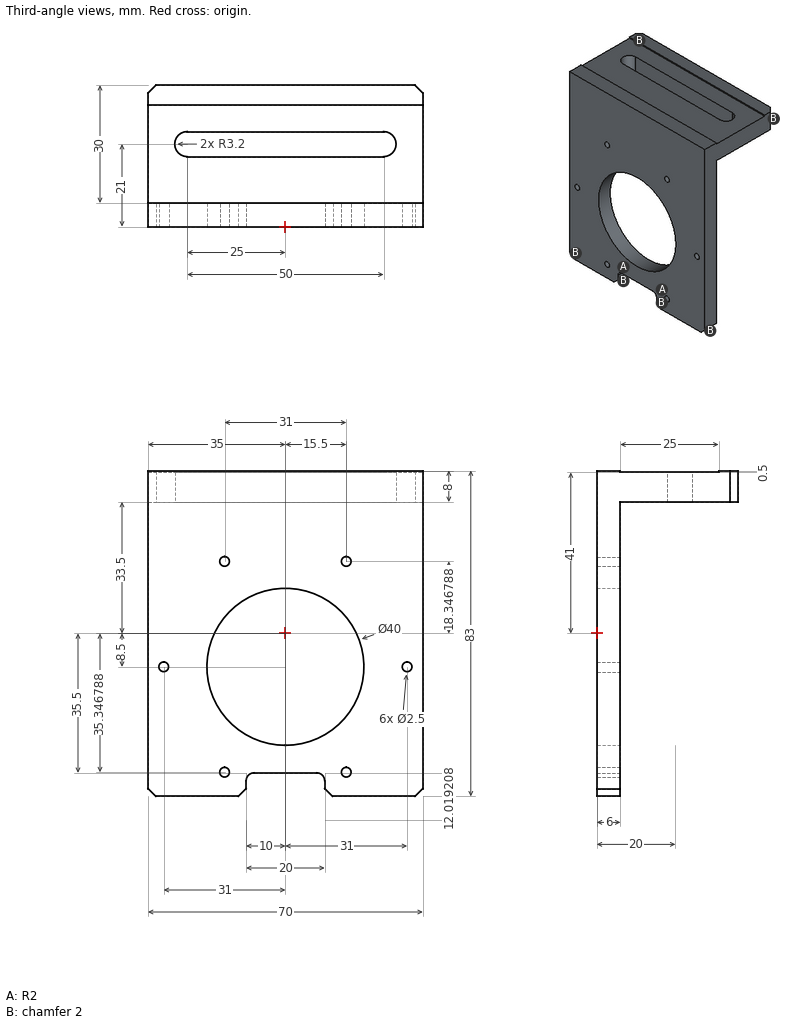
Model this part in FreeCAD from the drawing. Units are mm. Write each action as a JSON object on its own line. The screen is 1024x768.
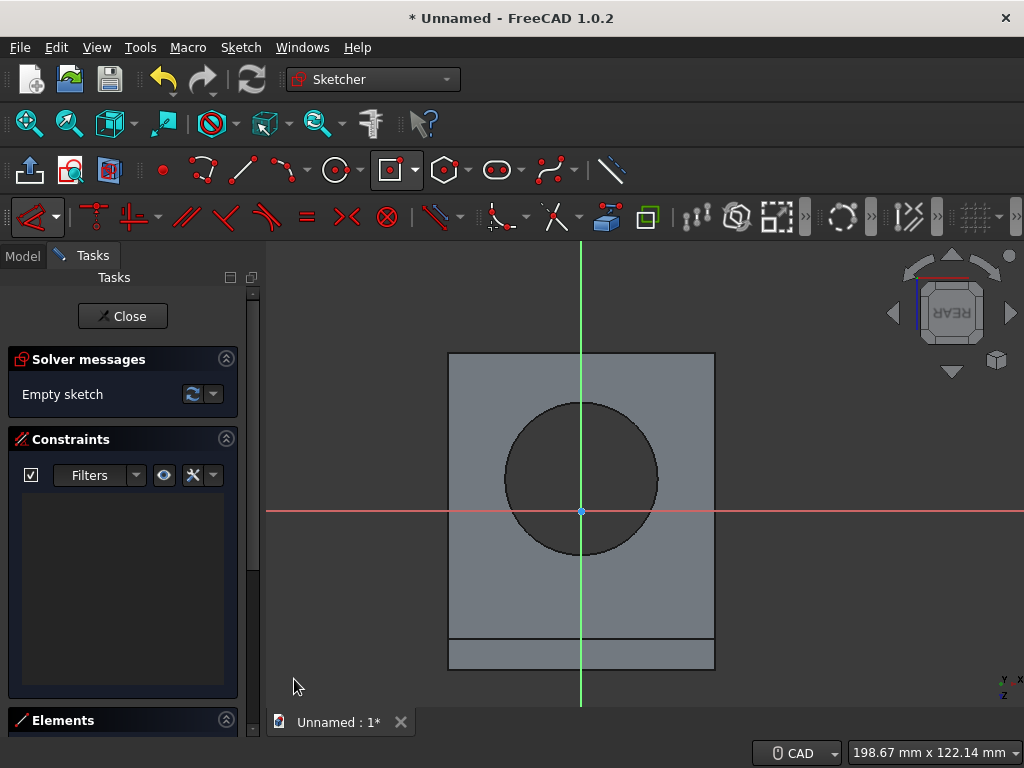
{"action": "scroll", "coordinate": [591, 312], "scroll_direction": "up", "scroll_amount": 2}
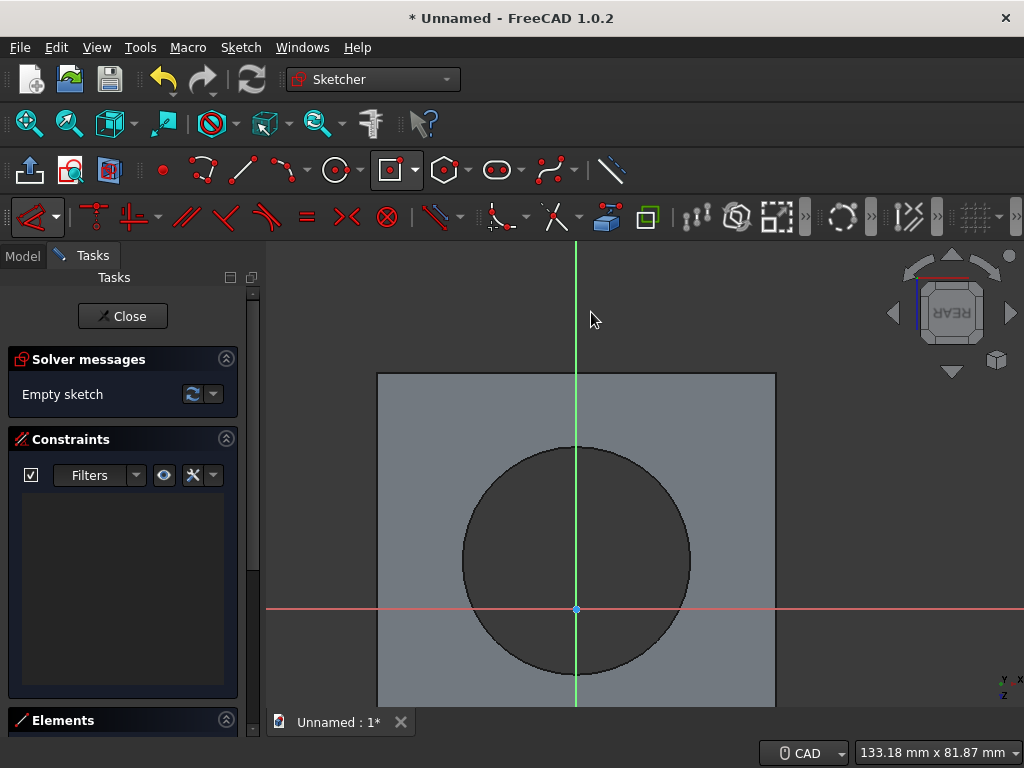
{"action": "left_click", "coordinate": [418, 170]}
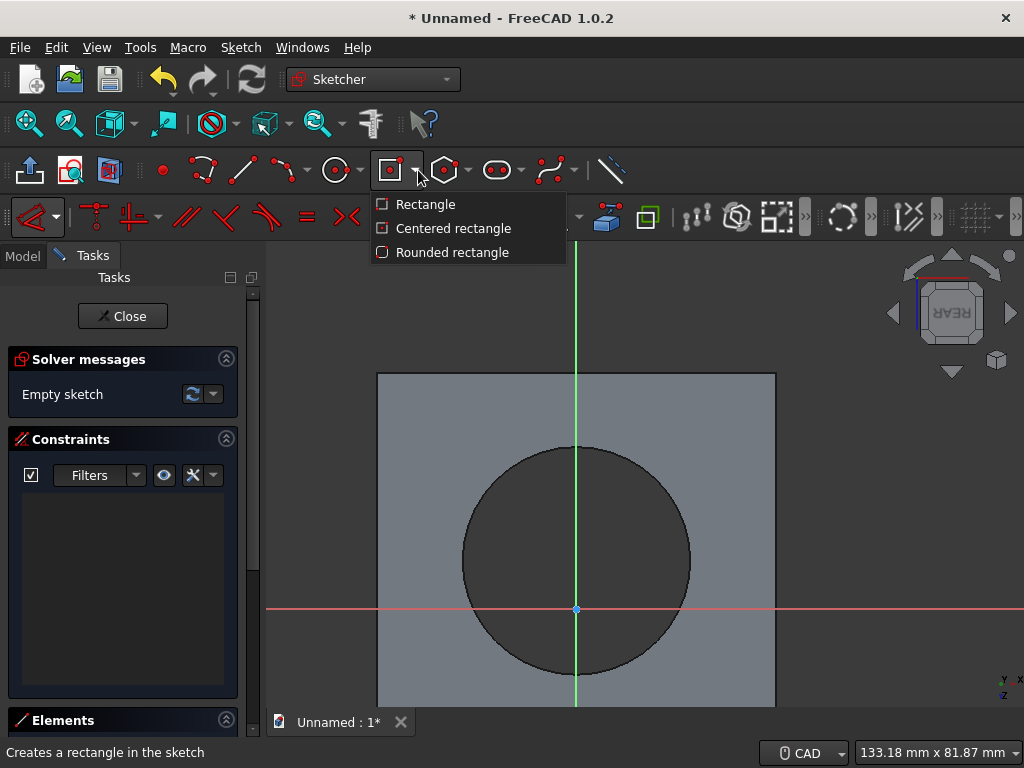
{"action": "left_click", "coordinate": [468, 204]}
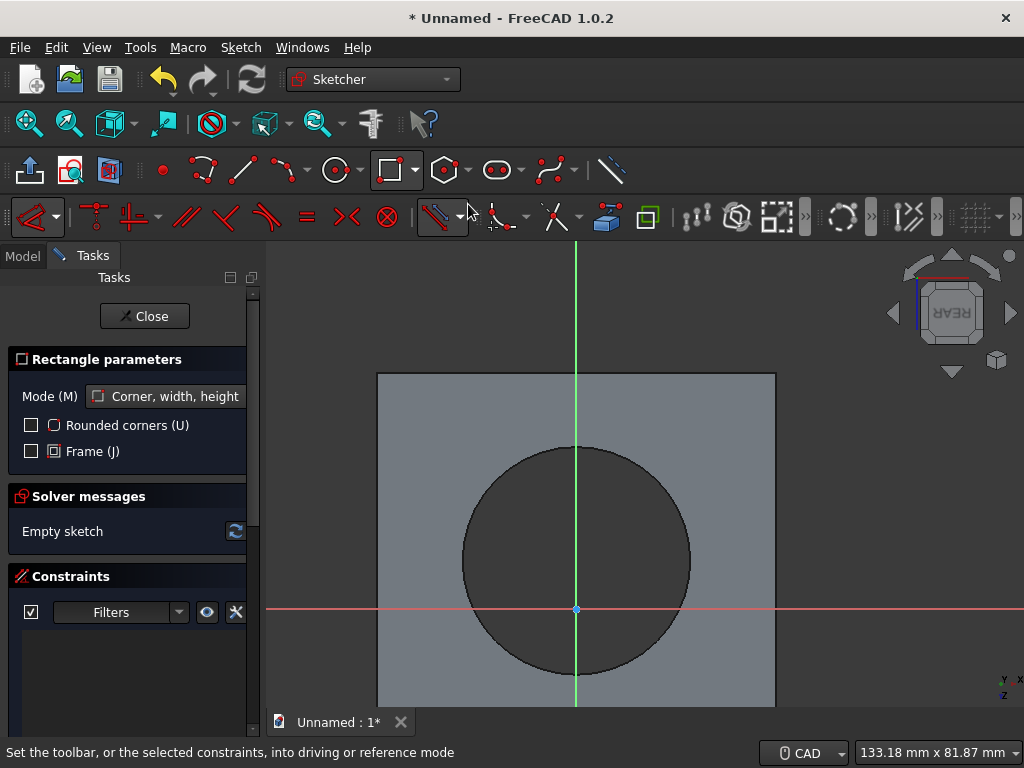
{"action": "left_click", "coordinate": [520, 339]}
{"action": "mouse_move", "coordinate": [633, 407]}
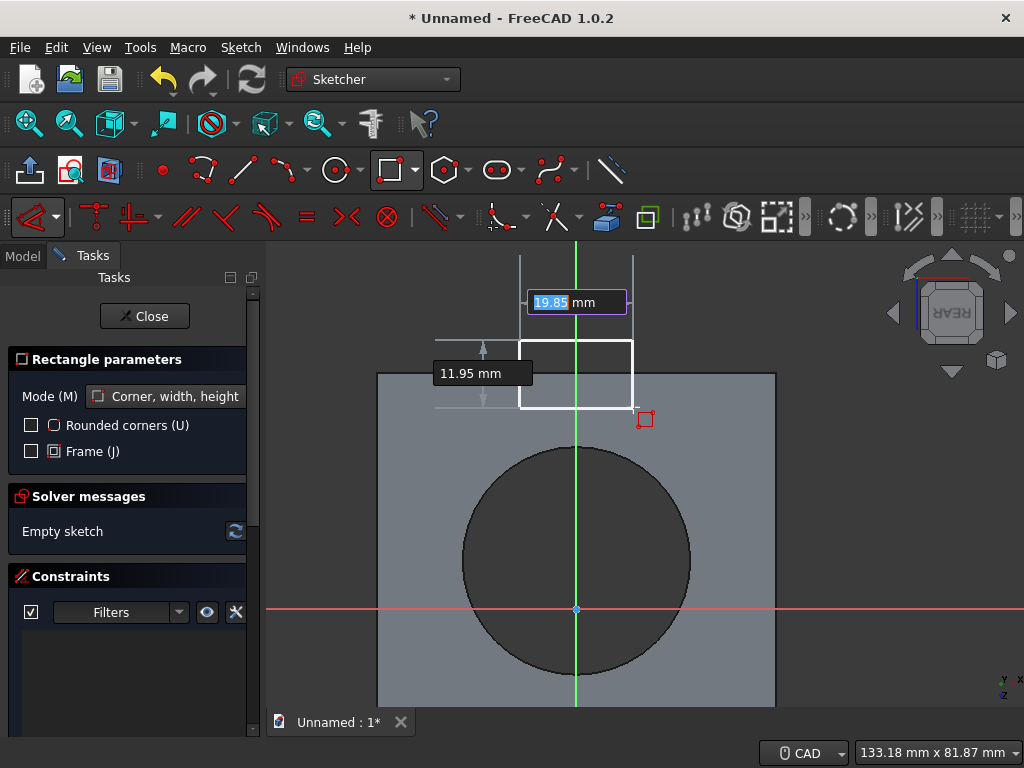
{"action": "type", "text": "20"}
{"action": "key", "text": "Tab"}
{"action": "type", "text": "12.019208"}
{"action": "key", "text": "Return"}
{"action": "key", "text": "Escape"}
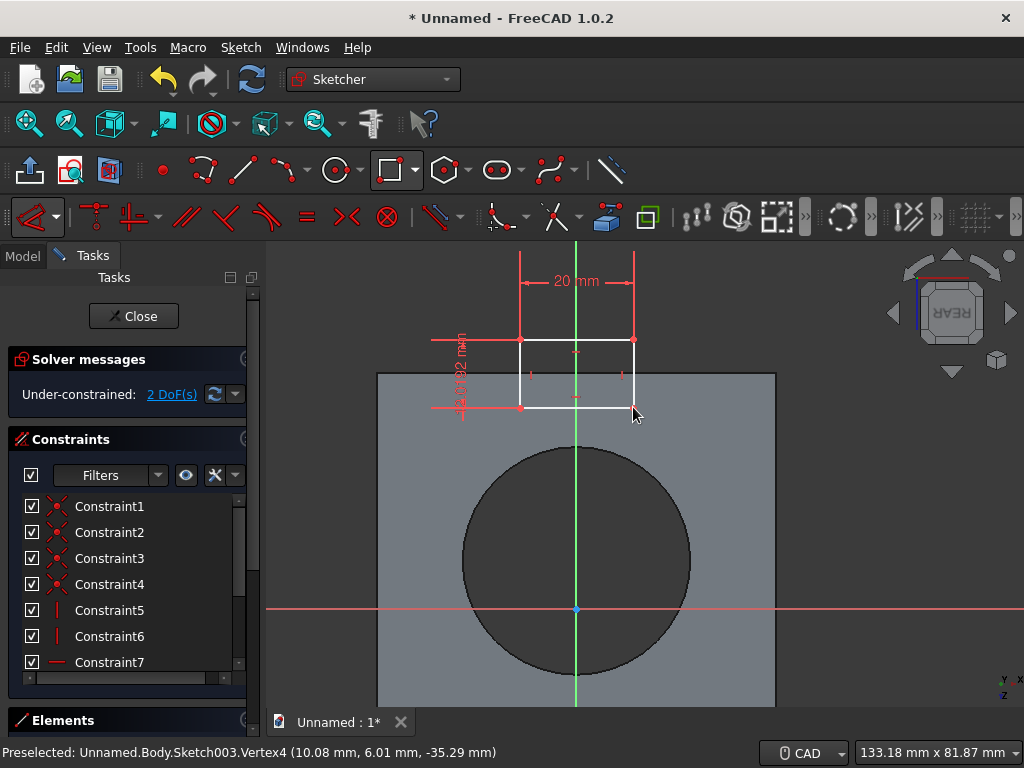
{"action": "left_click", "coordinate": [520, 340]}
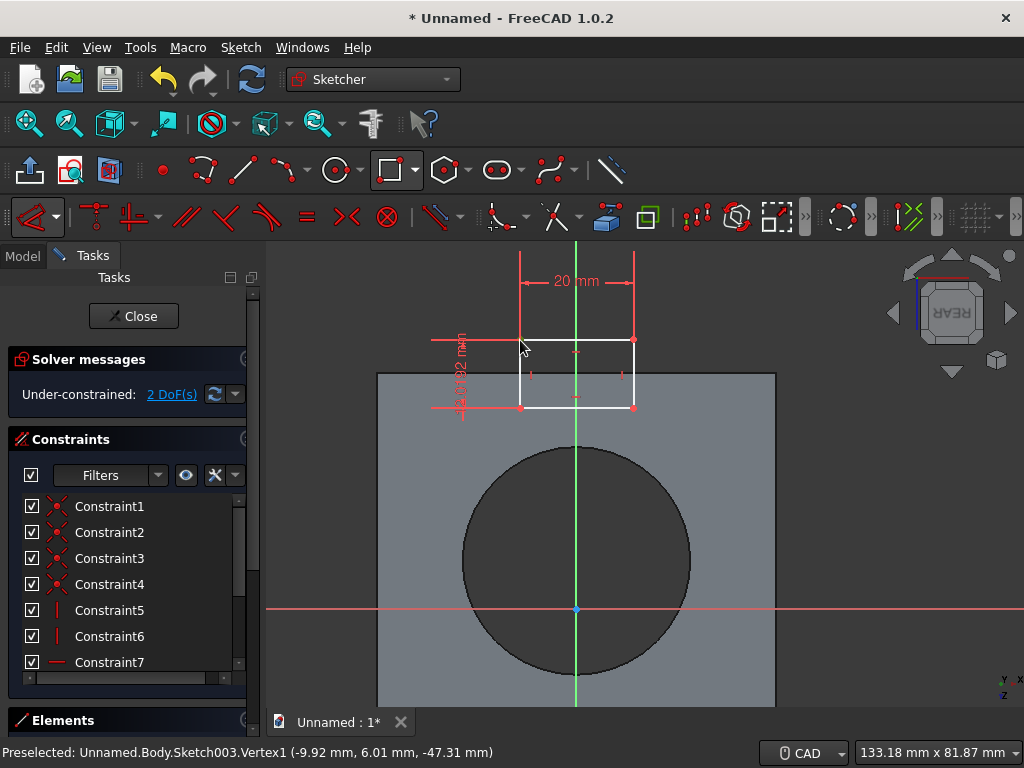
{"action": "key", "text": "l"}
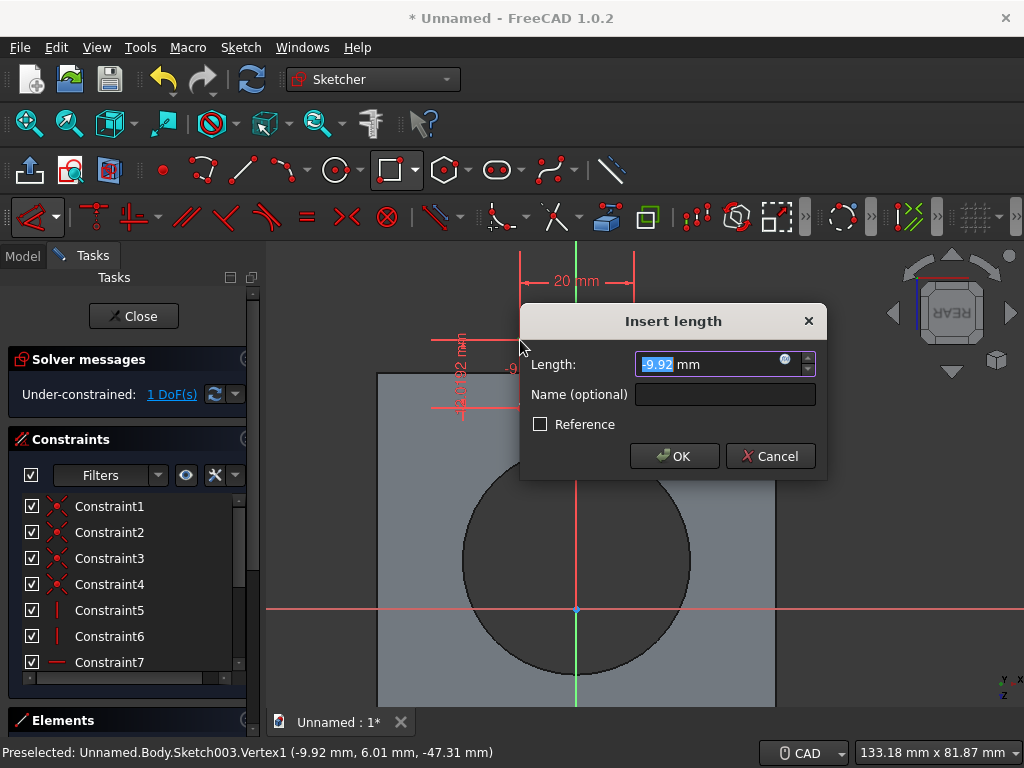
{"action": "type", "text": "-10"}
{"action": "key", "text": "Return"}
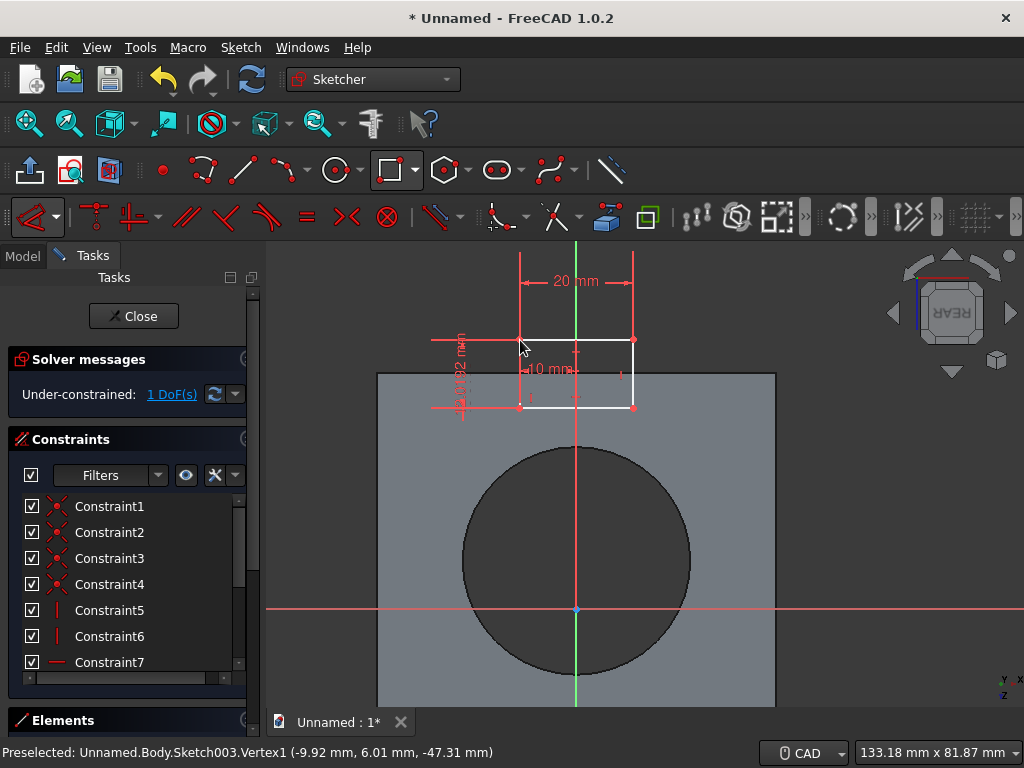
{"action": "left_click", "coordinate": [520, 408]}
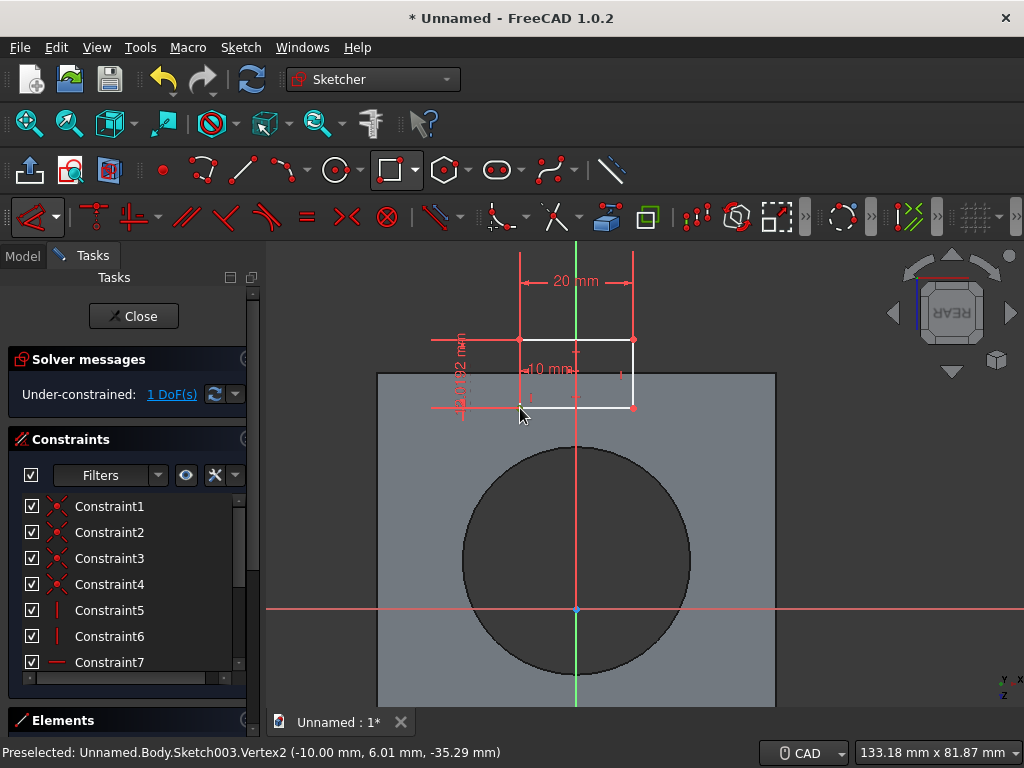
{"action": "left_click", "coordinate": [58, 218]}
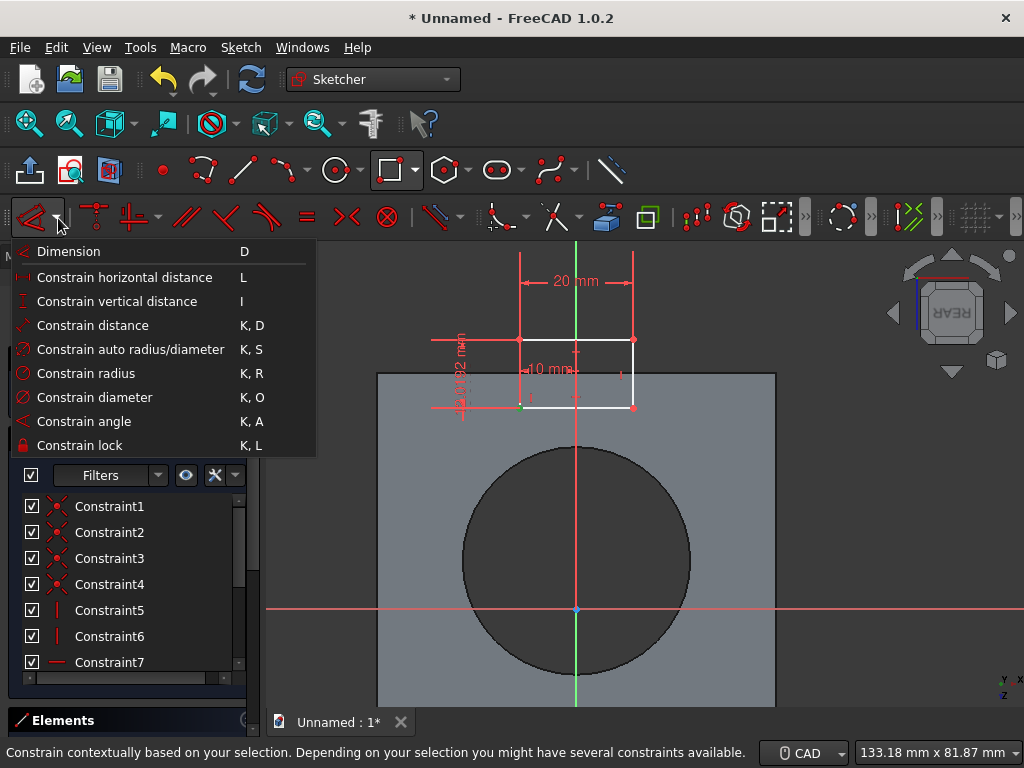
{"action": "left_click", "coordinate": [164, 301]}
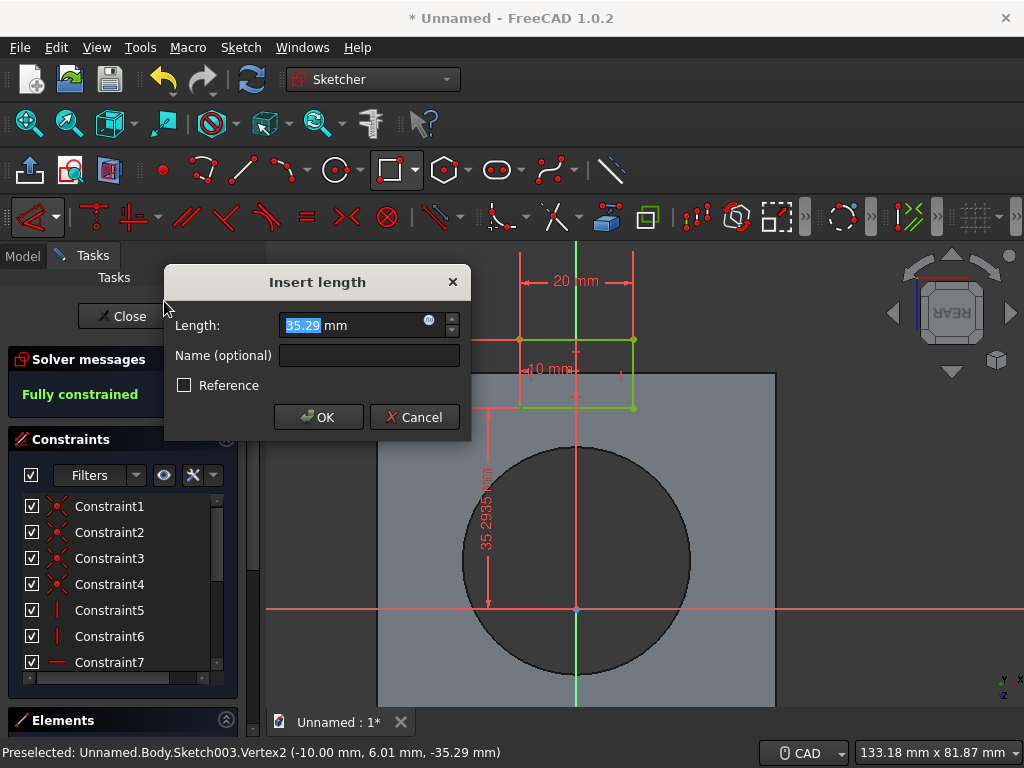
{"action": "type", "text": "35.5"}
{"action": "key", "text": "Return"}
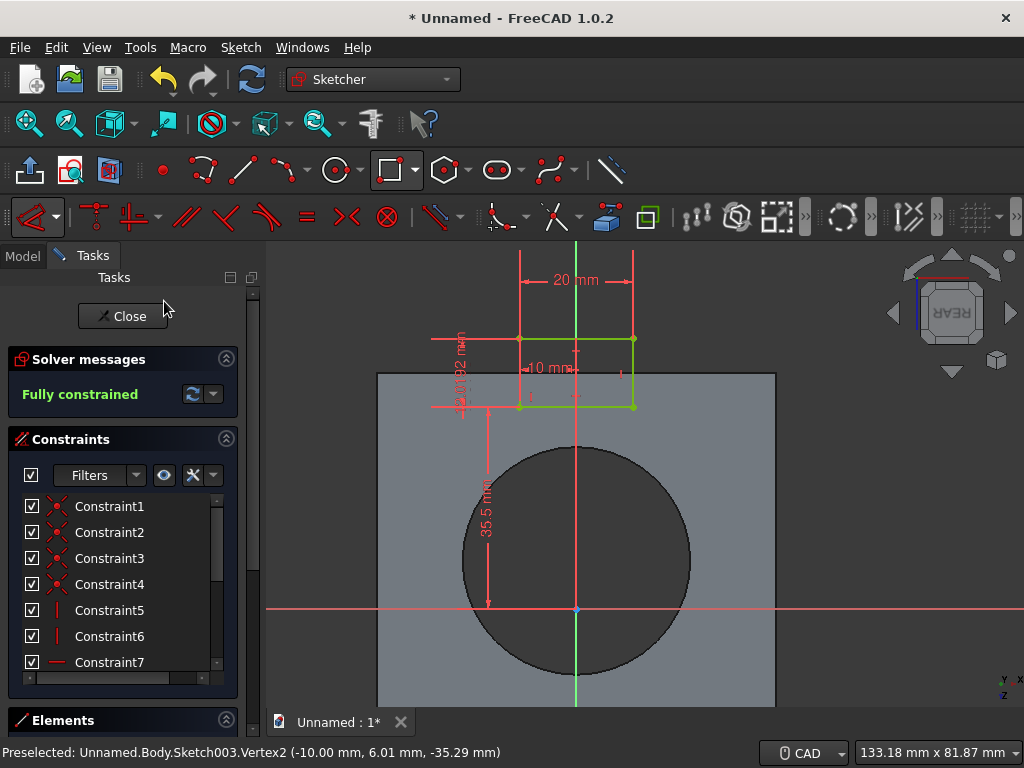
{"action": "left_click", "coordinate": [123, 316]}